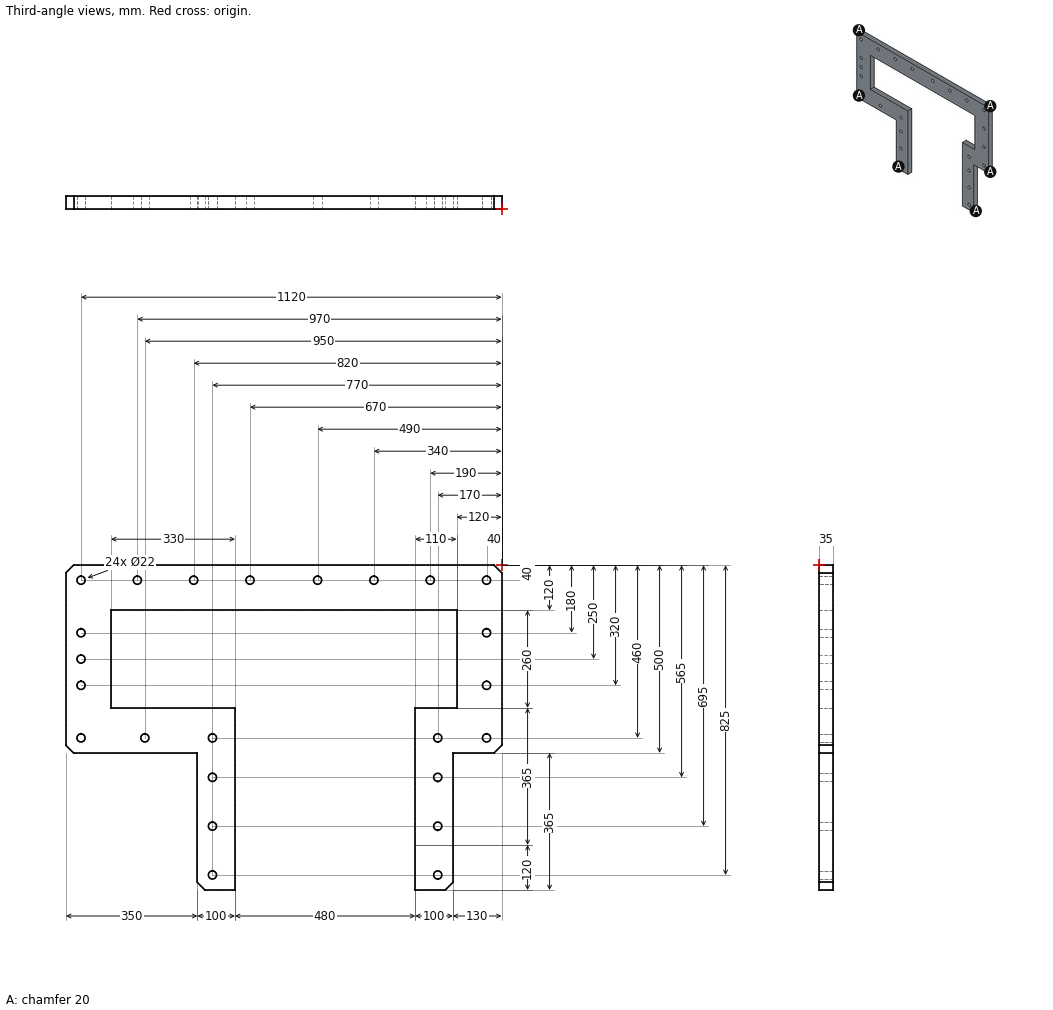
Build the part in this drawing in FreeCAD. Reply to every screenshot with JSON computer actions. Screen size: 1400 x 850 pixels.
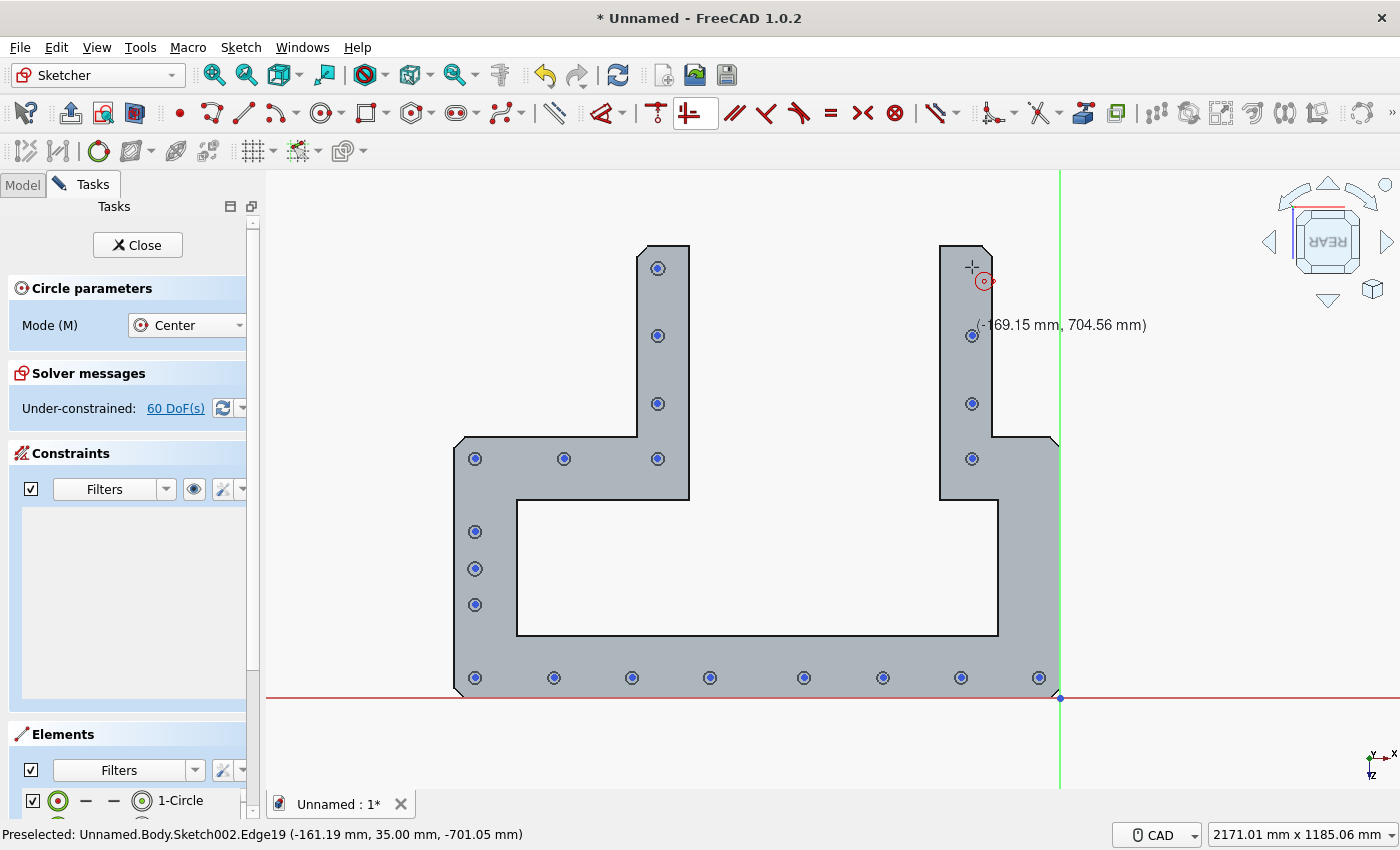
{"action": "left_click", "coordinate": [972, 267]}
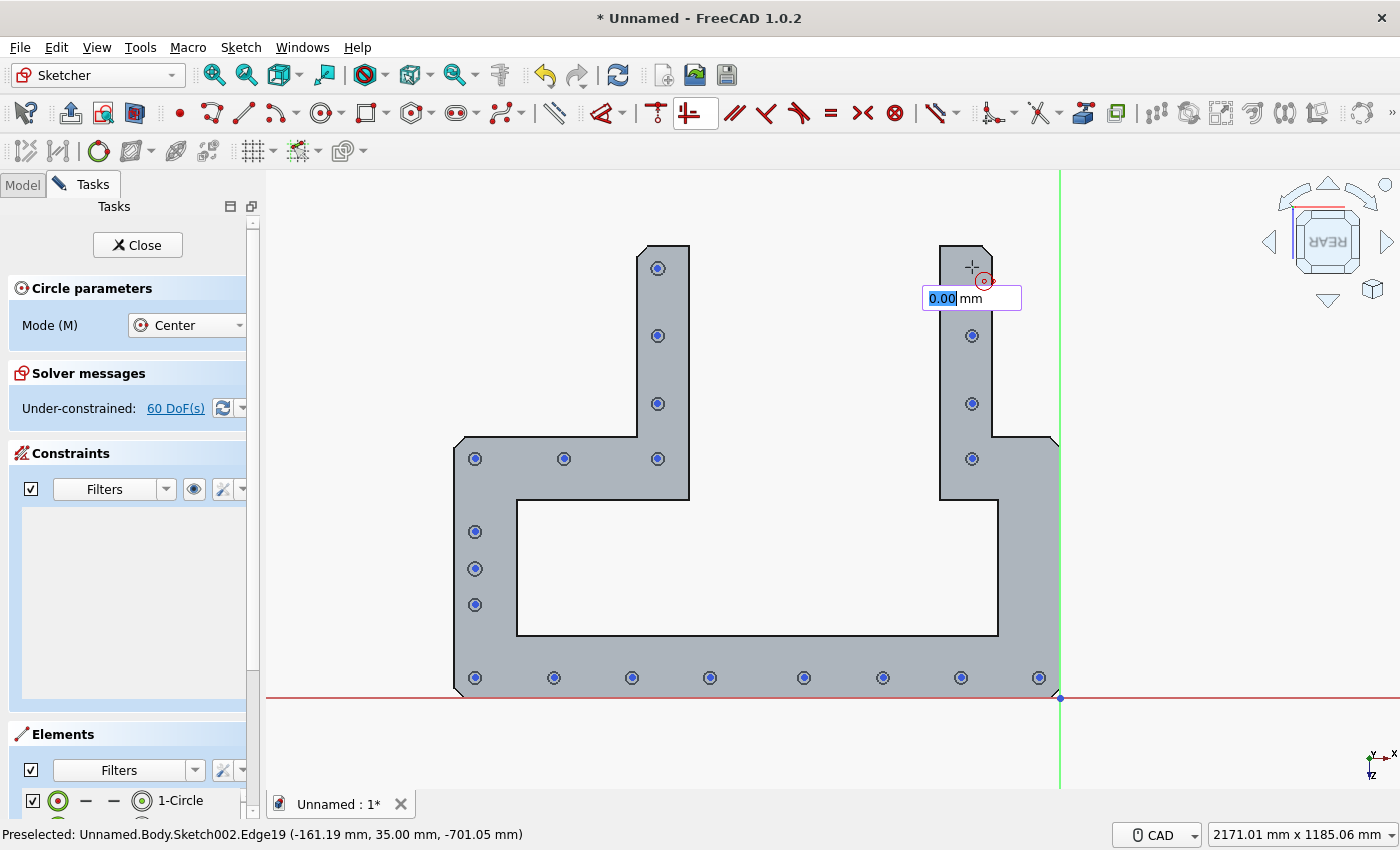
{"action": "scroll", "coordinate": [976, 263], "scroll_direction": "up", "scroll_amount": 6}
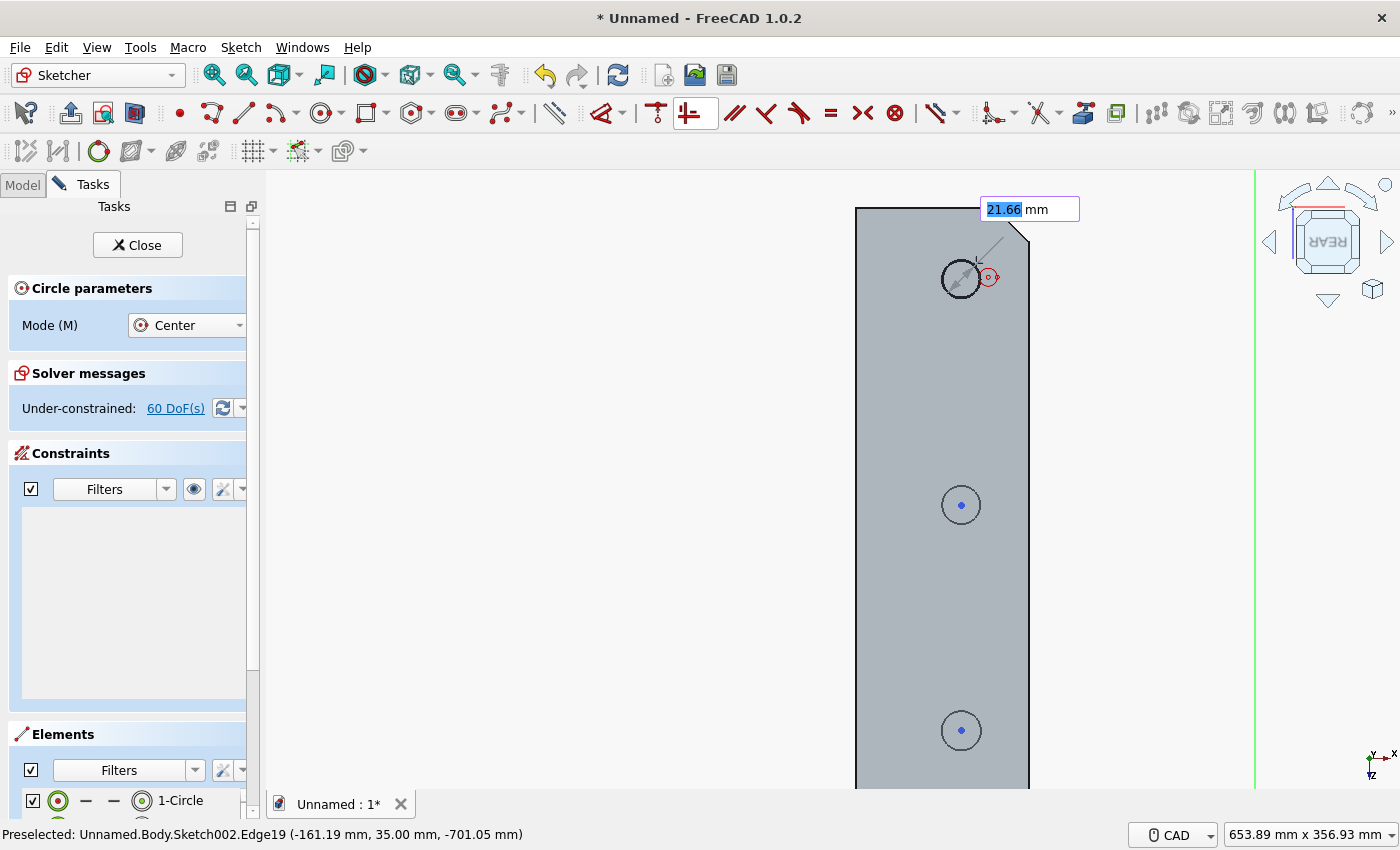
{"action": "left_click", "coordinate": [973, 264]}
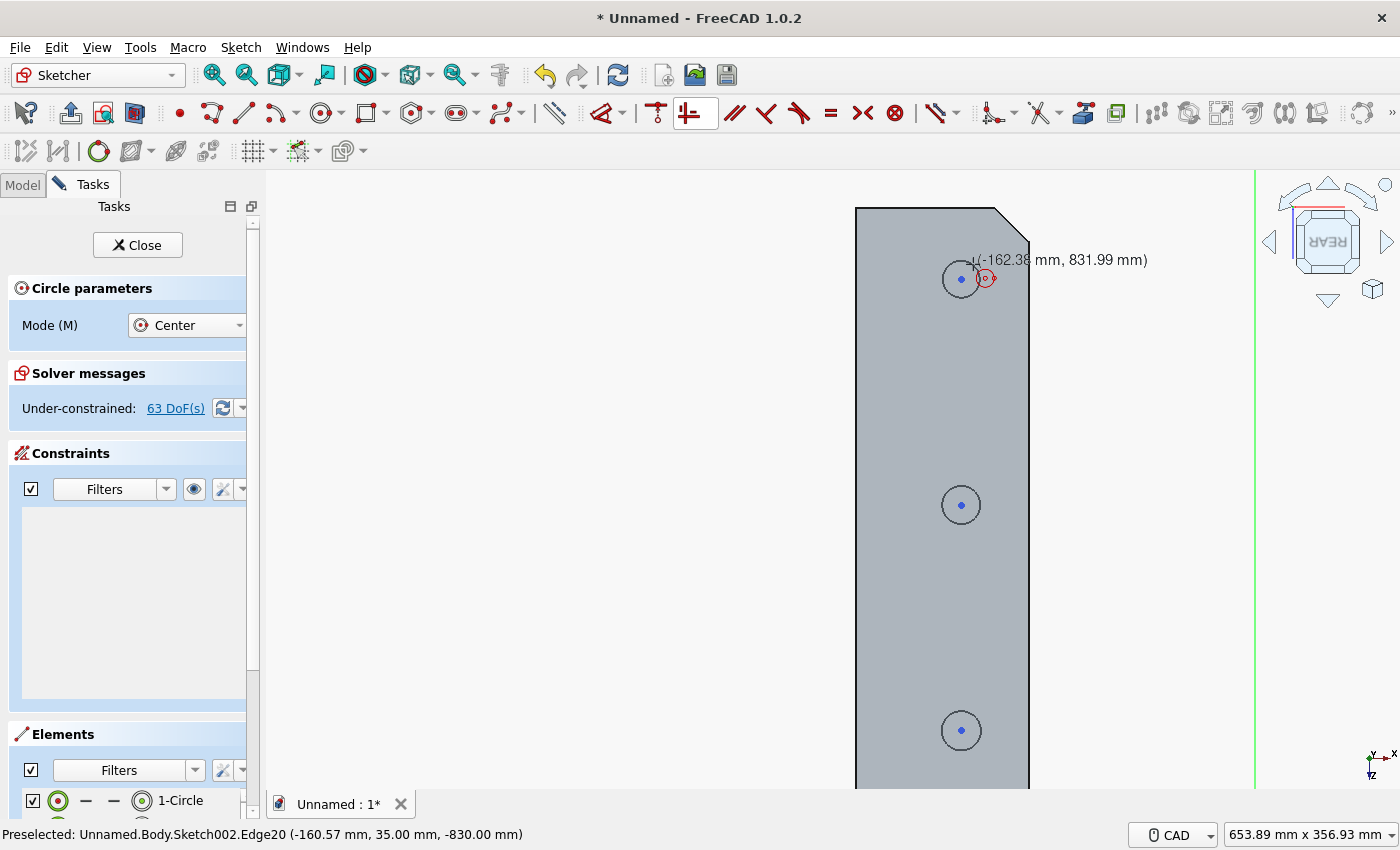
{"action": "scroll", "coordinate": [976, 263], "scroll_direction": "down", "scroll_amount": 6}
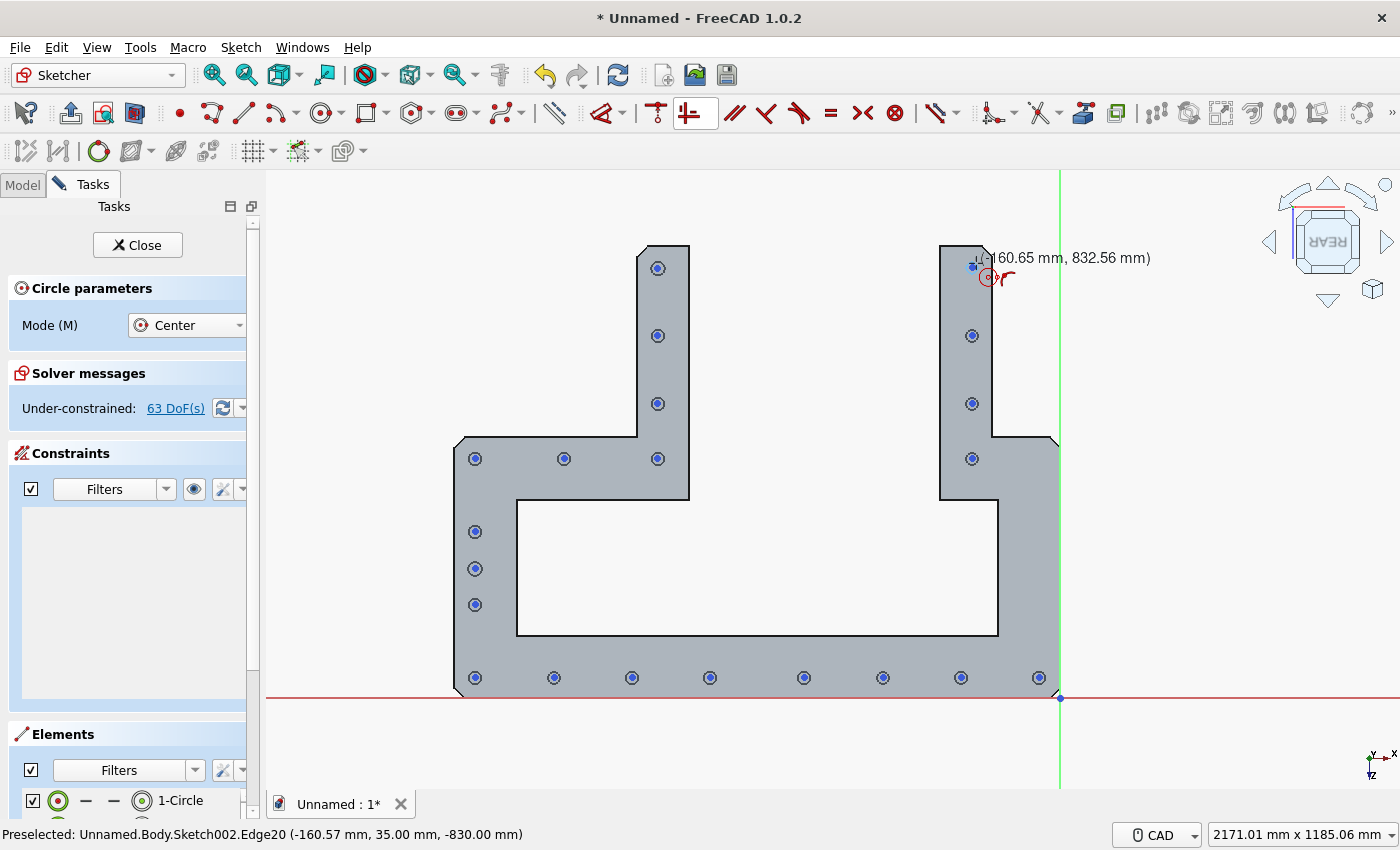
{"action": "scroll", "coordinate": [1039, 458], "scroll_direction": "up", "scroll_amount": 7}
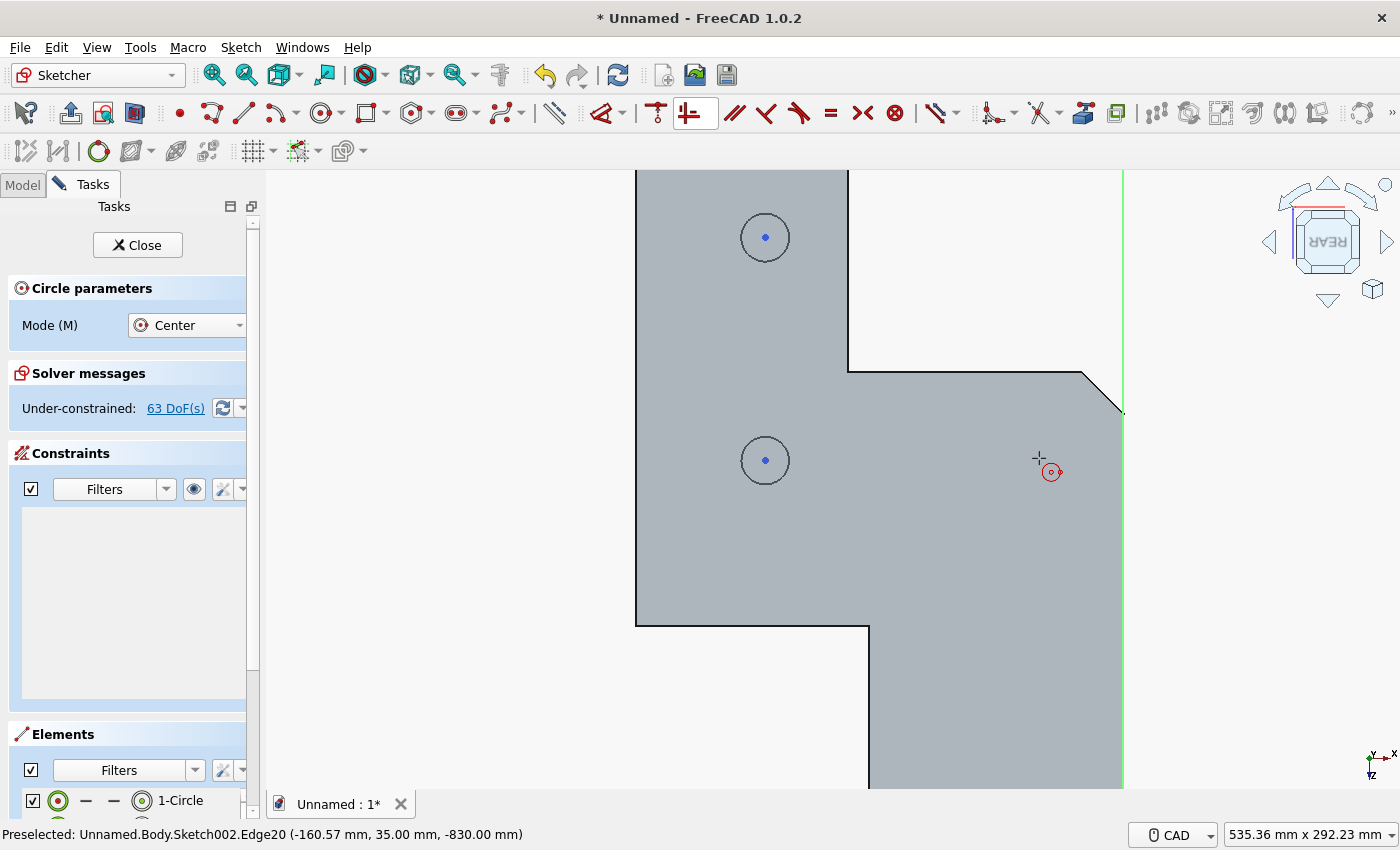
{"action": "scroll", "coordinate": [1039, 458], "scroll_direction": "down", "scroll_amount": 7}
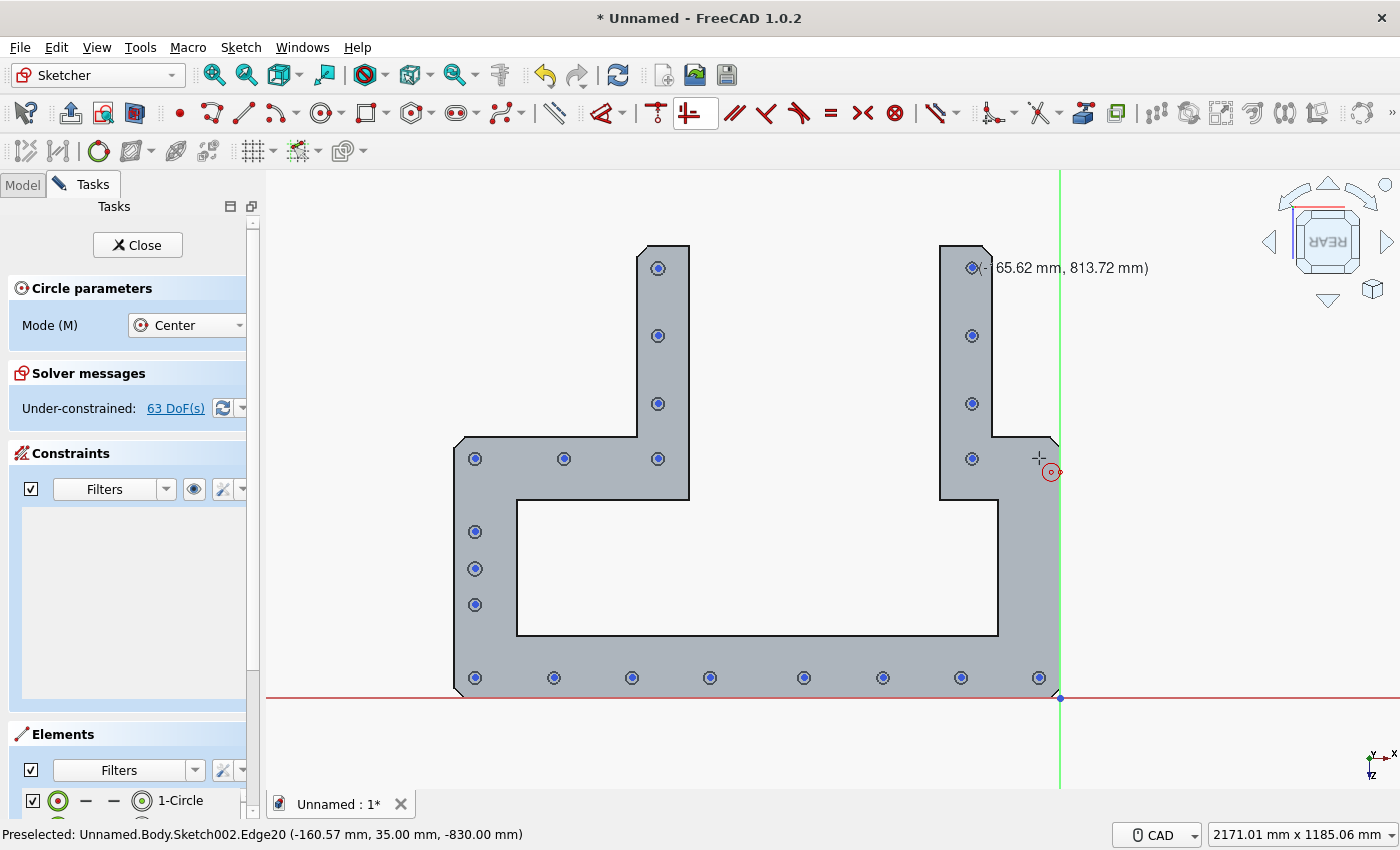
{"action": "left_click", "coordinate": [1039, 458]}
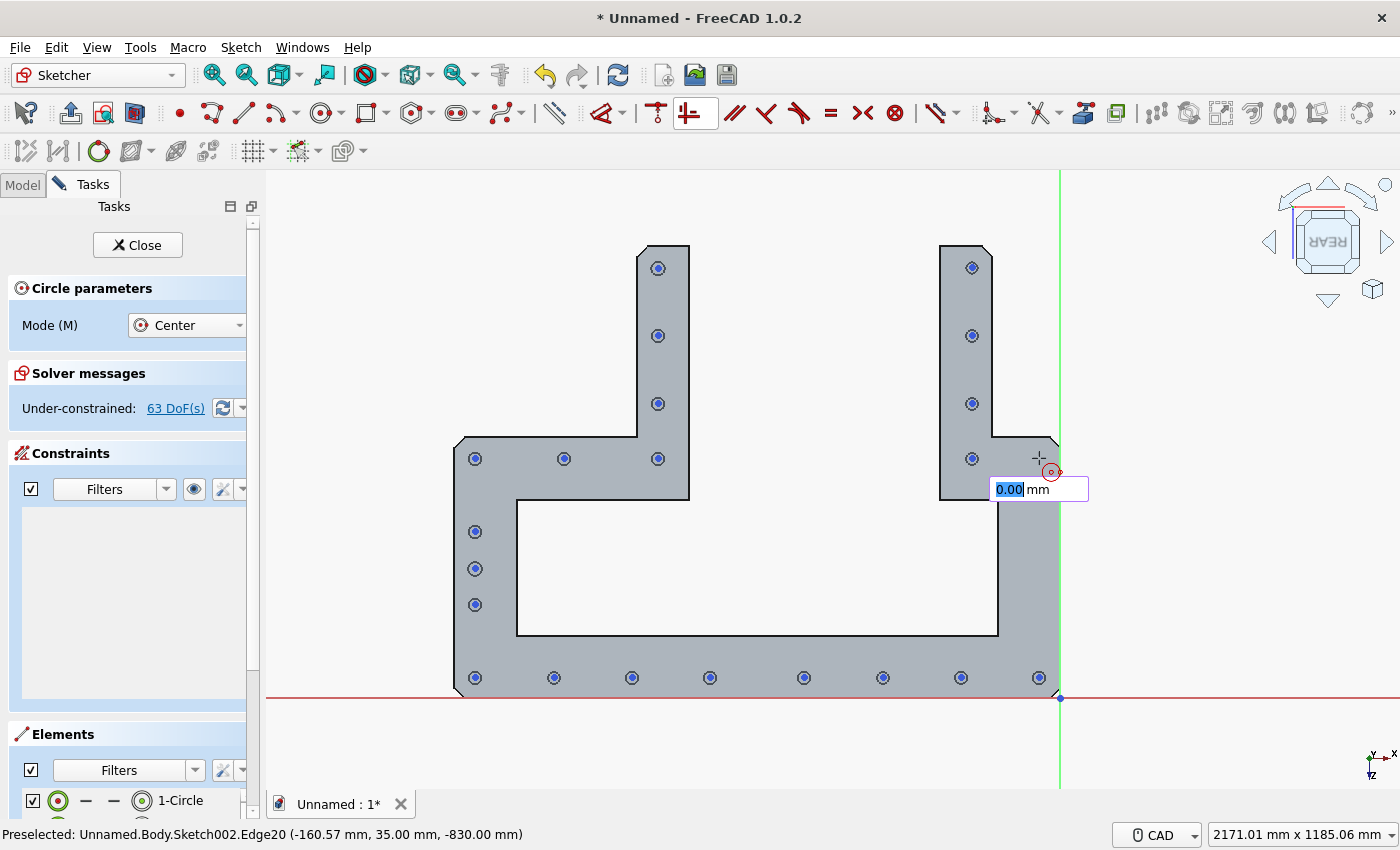
{"action": "scroll", "coordinate": [1044, 454], "scroll_direction": "up", "scroll_amount": 6}